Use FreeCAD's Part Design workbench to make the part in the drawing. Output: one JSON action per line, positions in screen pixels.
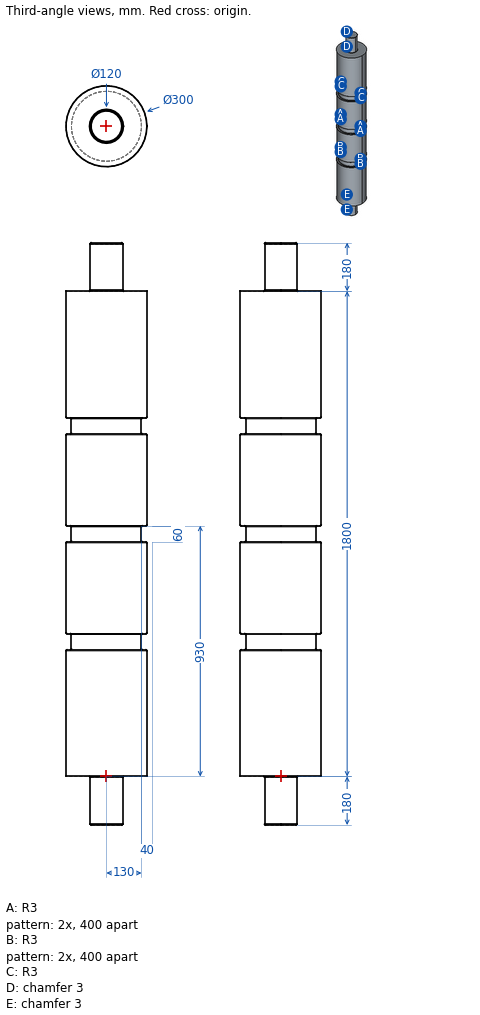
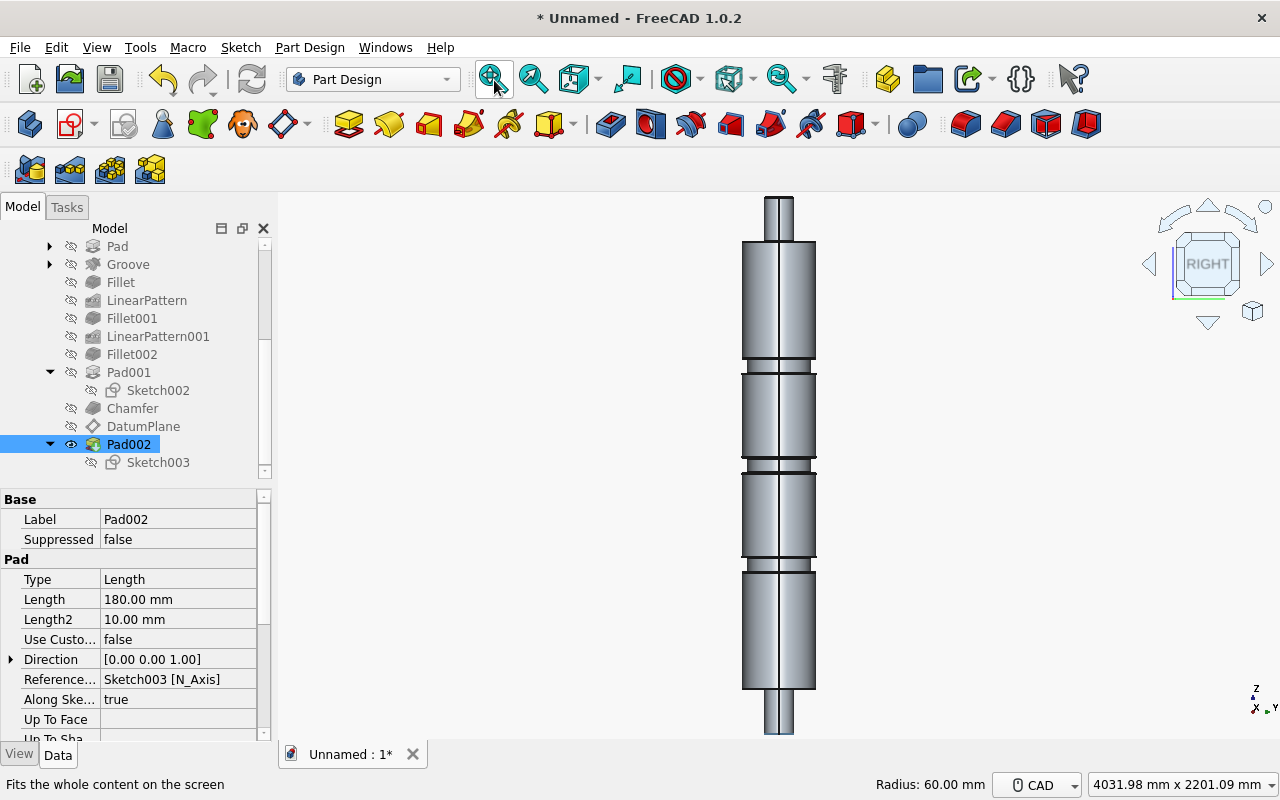
{"action": "key", "text": "5"}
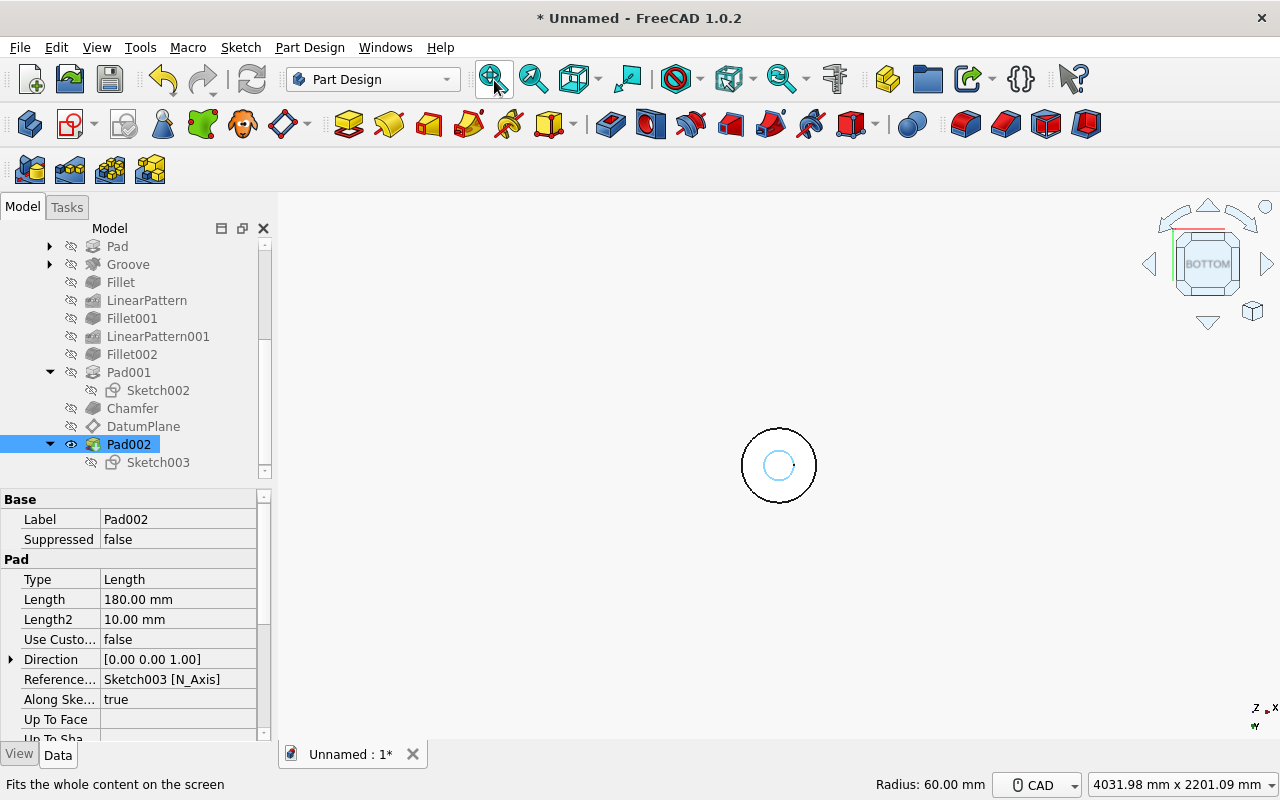
{"action": "left_click", "coordinate": [494, 80]}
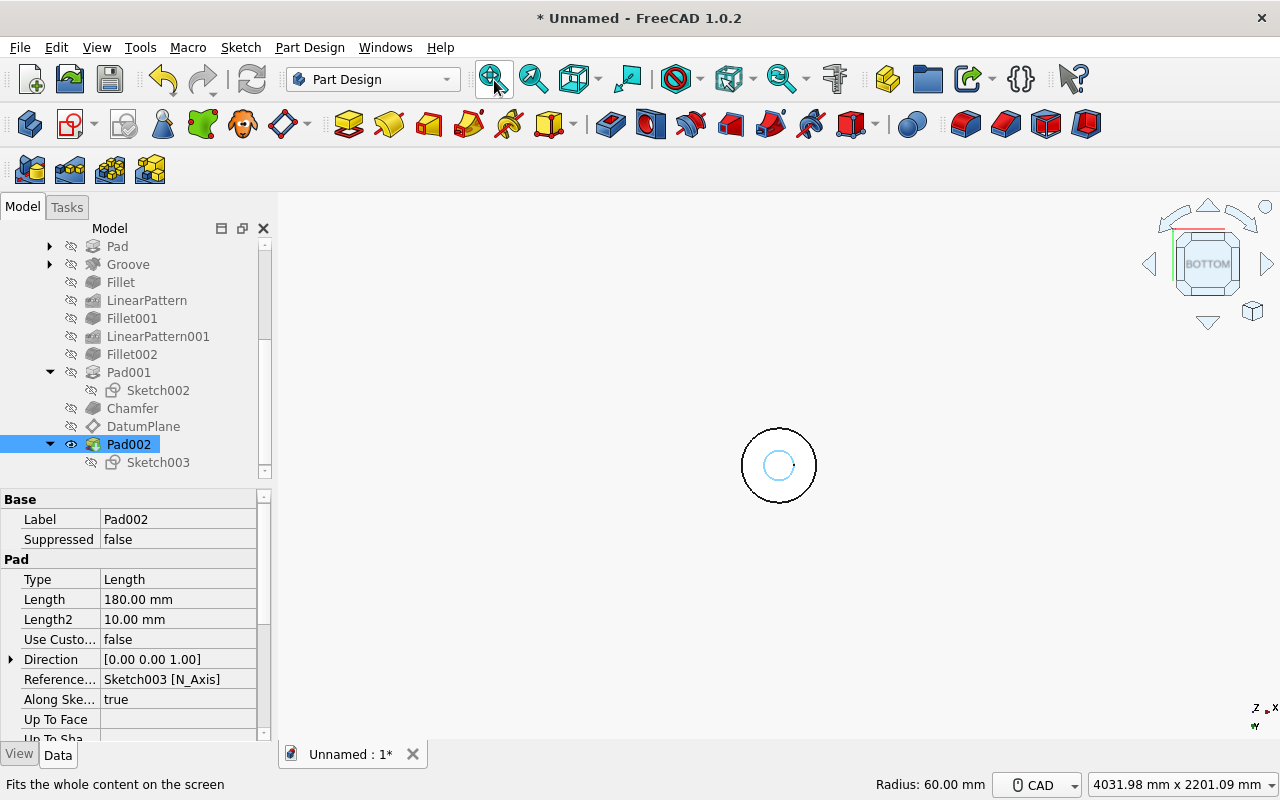
{"action": "key", "text": "4"}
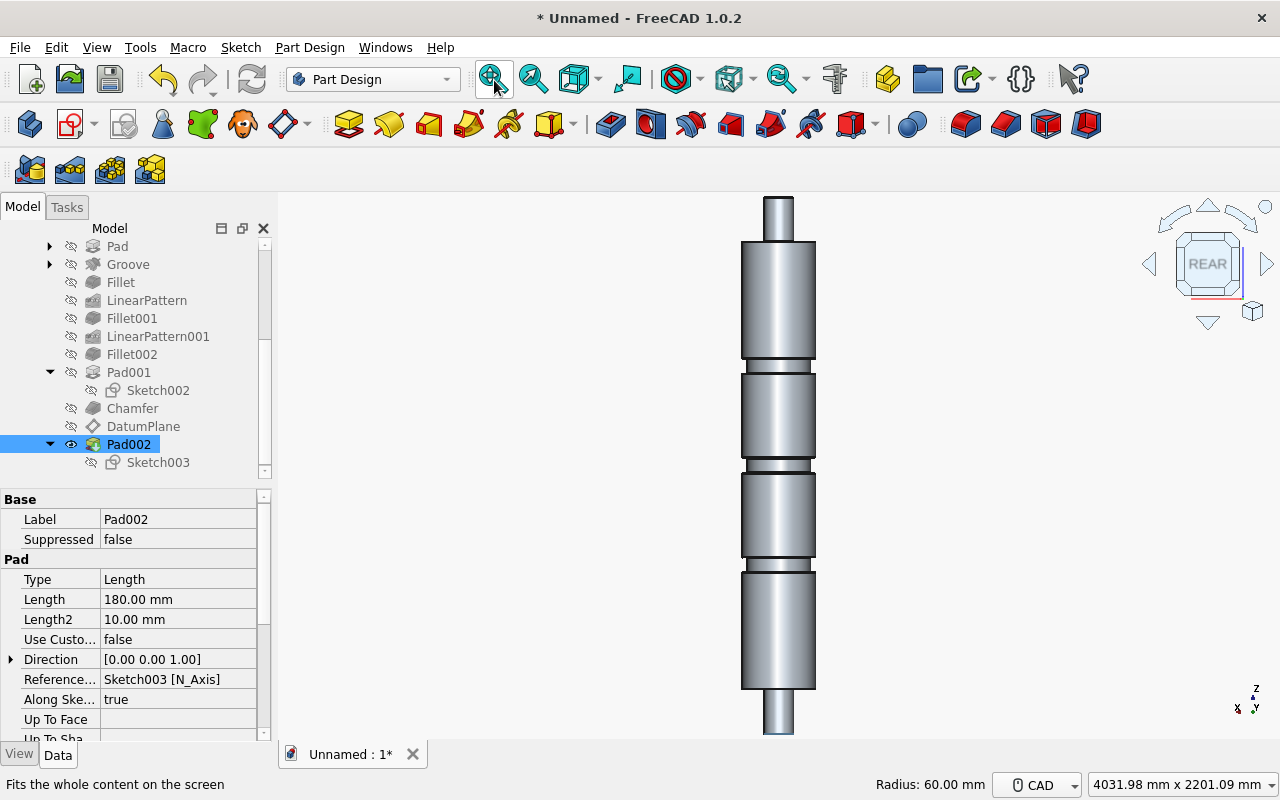
{"action": "key", "text": "6"}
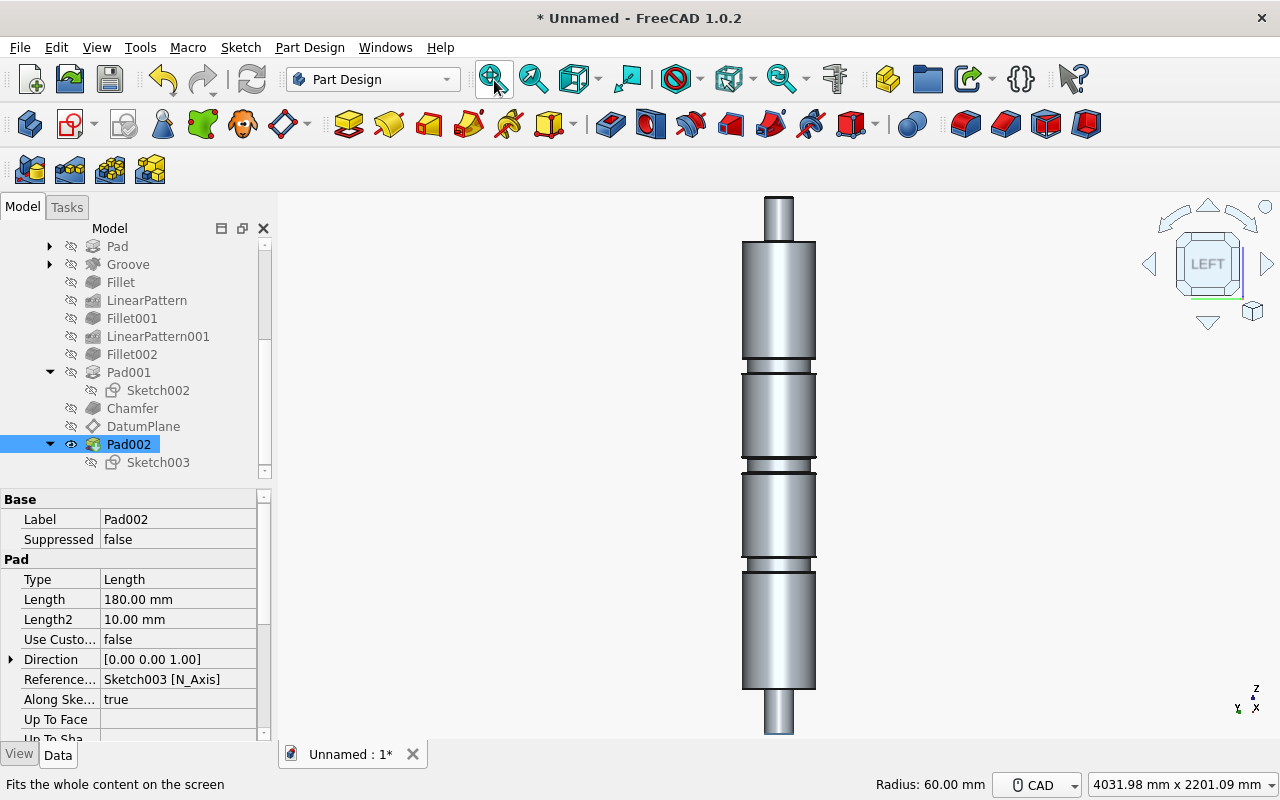
{"action": "key", "text": "v 3"}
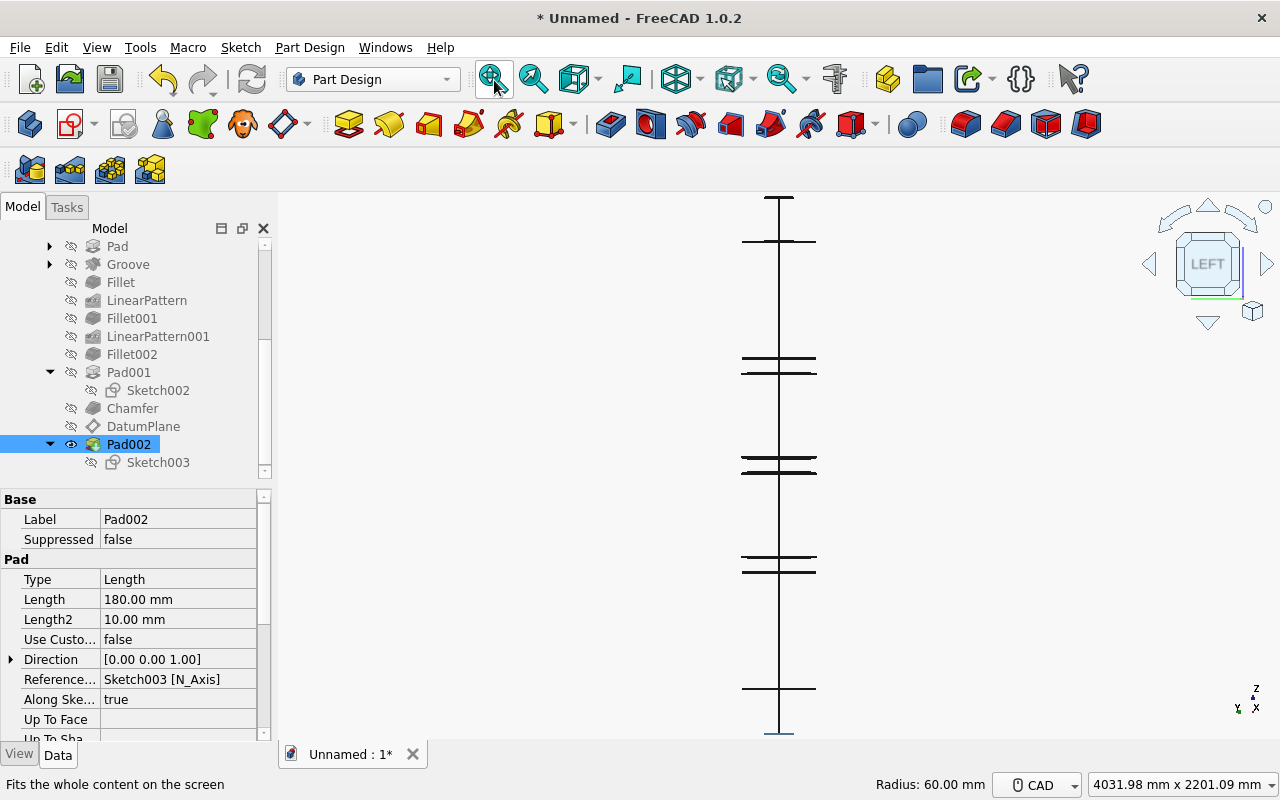
{"action": "key", "text": "0"}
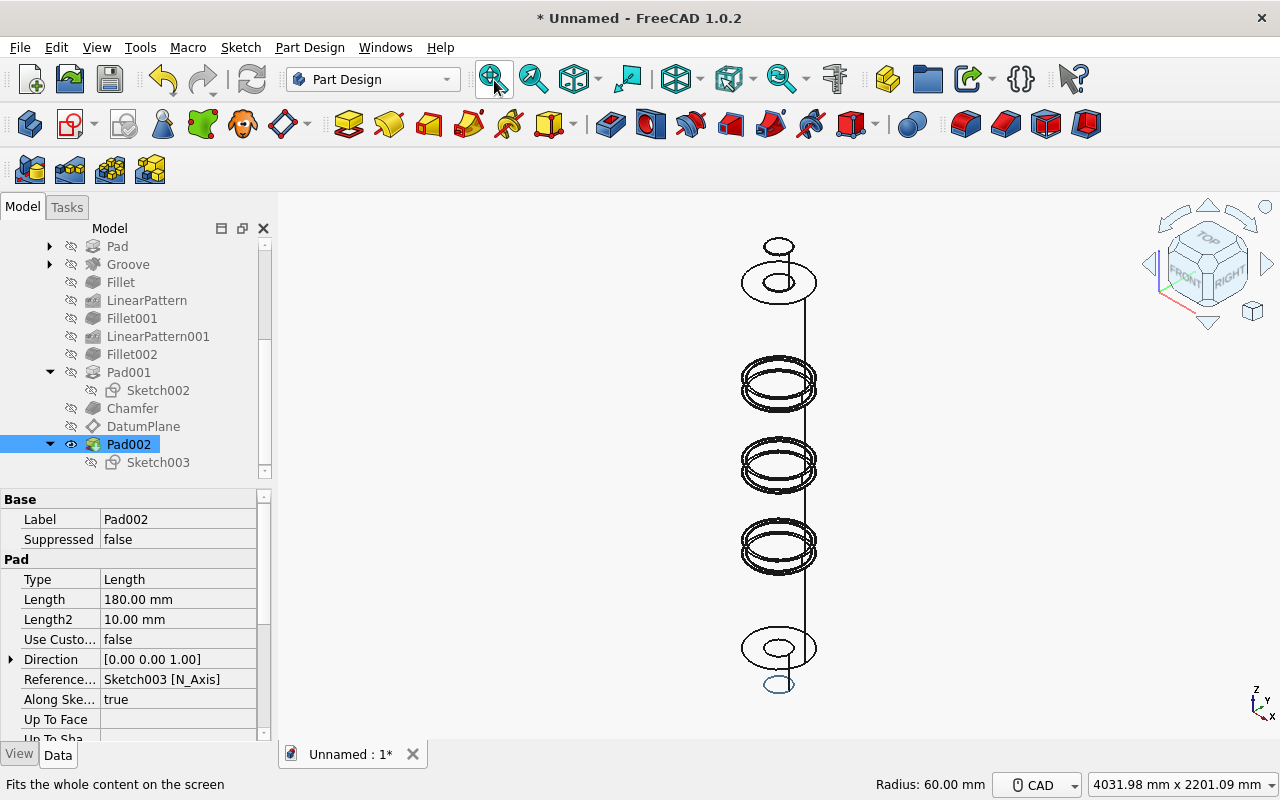
{"action": "left_click", "coordinate": [768, 641], "text": "ctrl"}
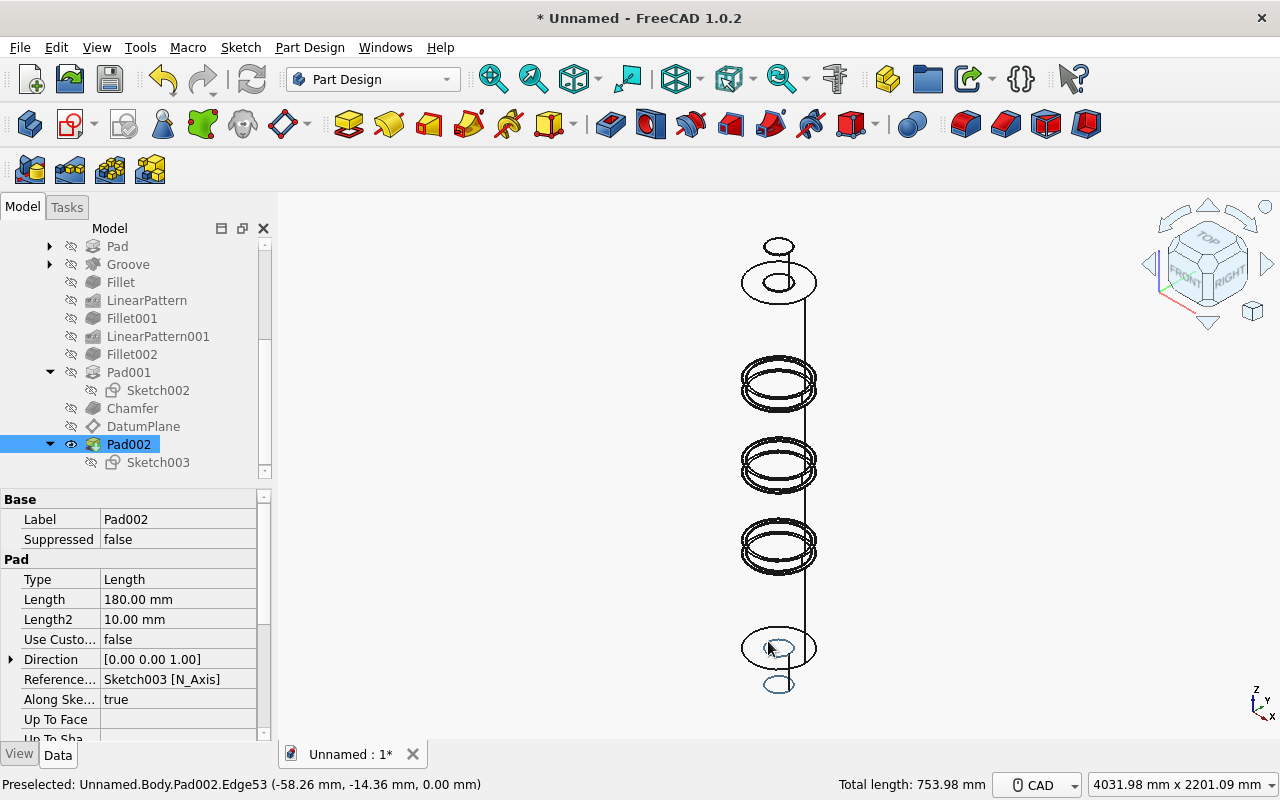
{"action": "key", "text": "v 1"}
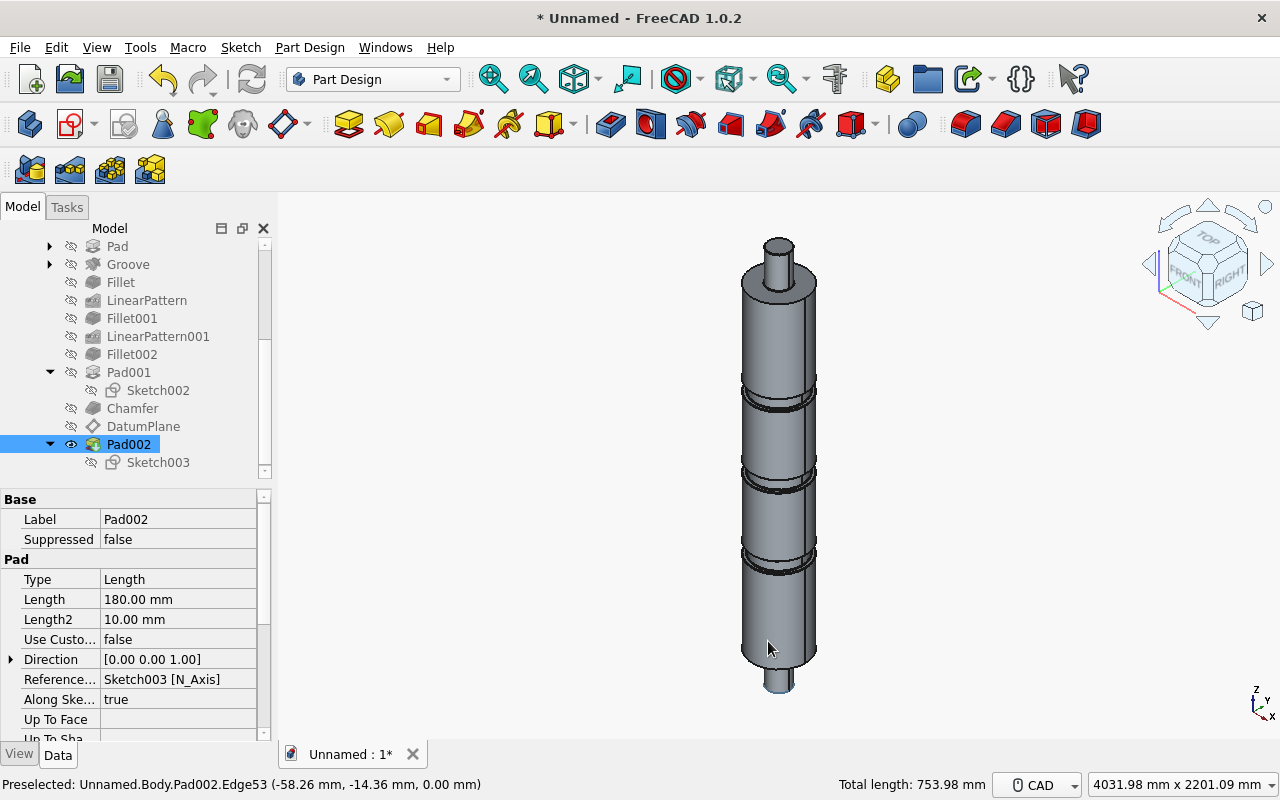
{"action": "left_click", "coordinate": [1006, 124]}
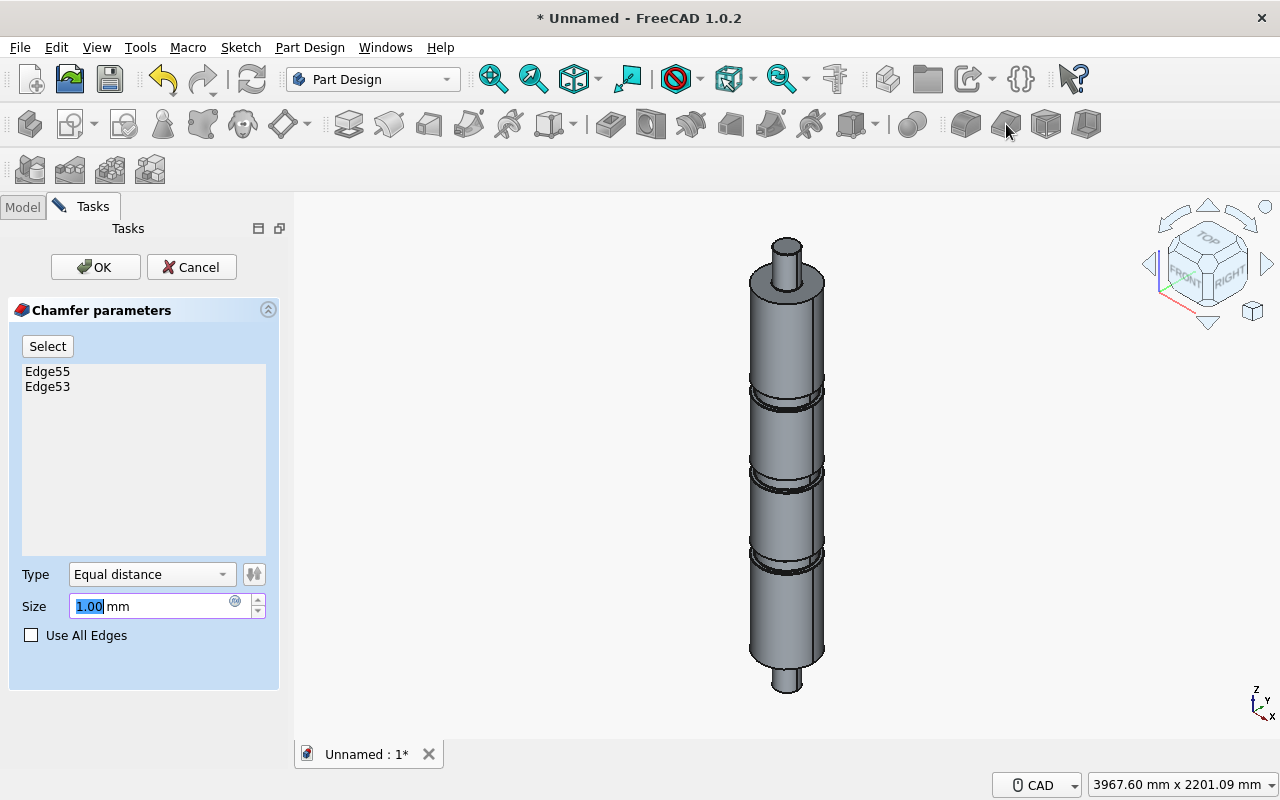
{"action": "type", "text": "3"}
{"action": "key", "text": "Tab"}